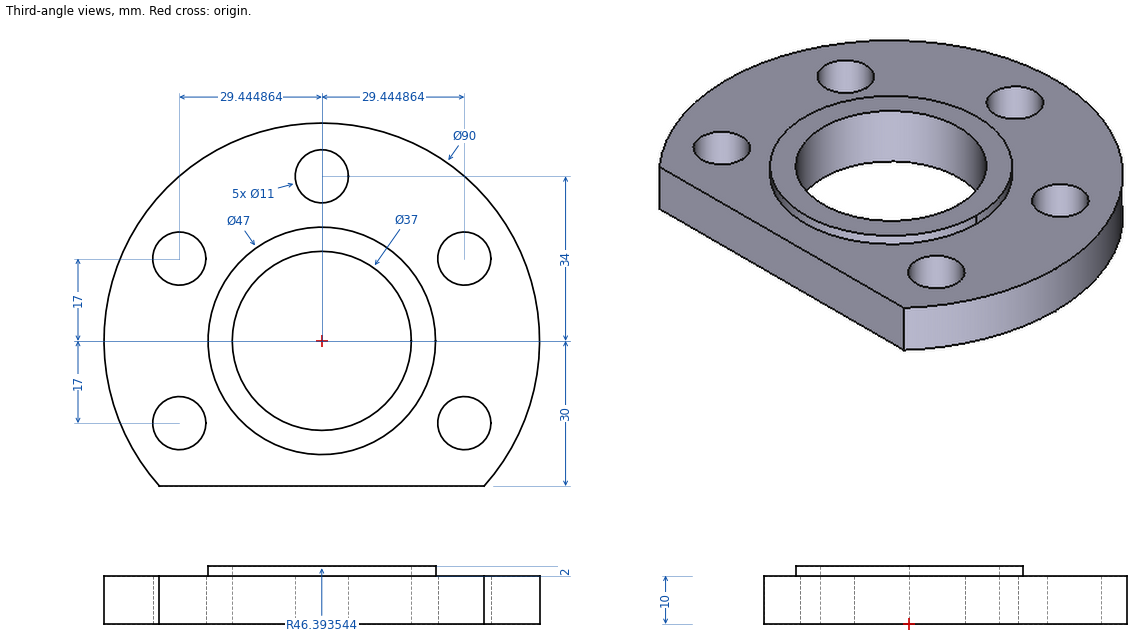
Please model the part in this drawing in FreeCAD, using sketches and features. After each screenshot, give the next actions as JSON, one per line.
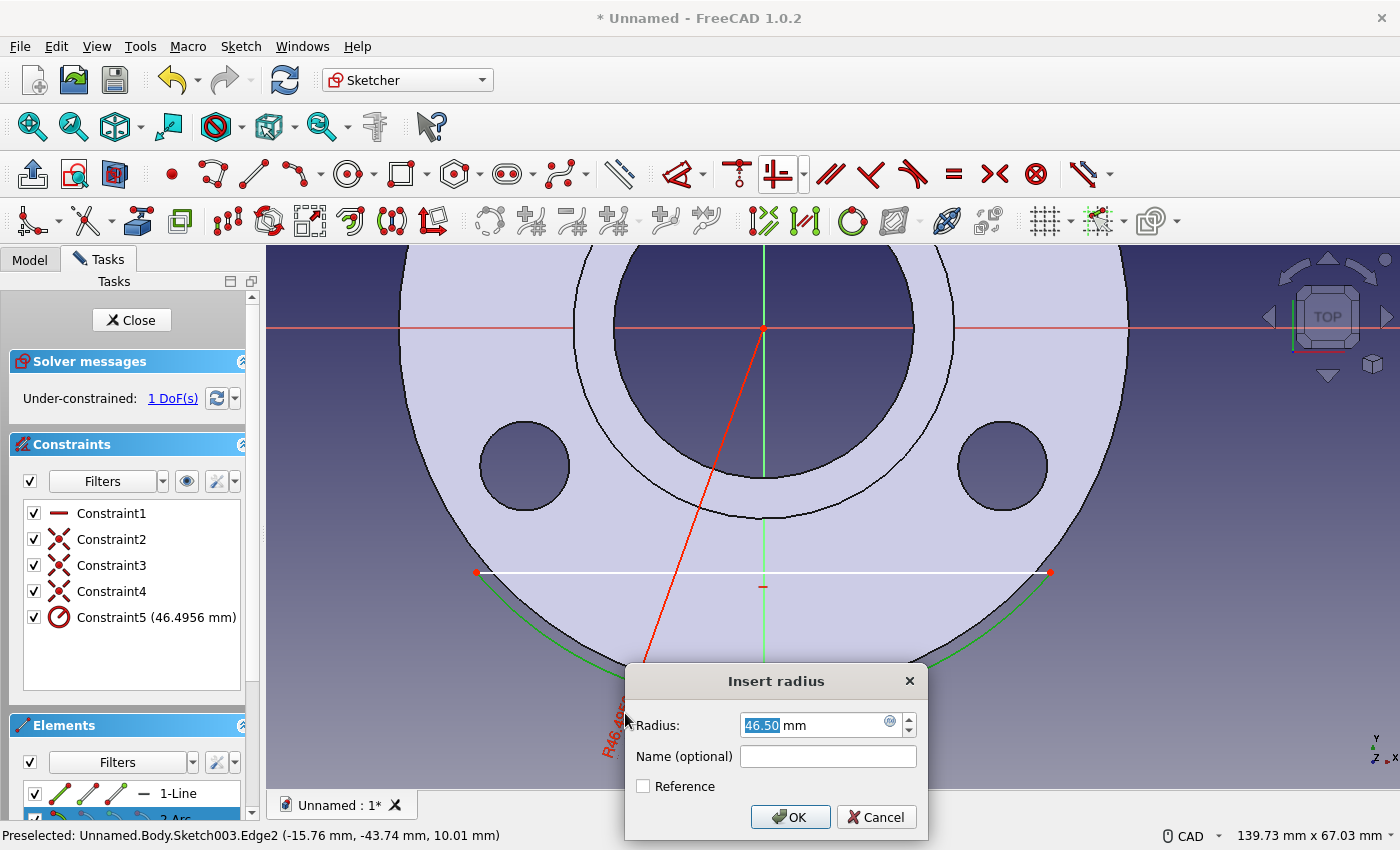
{"action": "type", "text": "46.393544"}
{"action": "key", "text": "Return"}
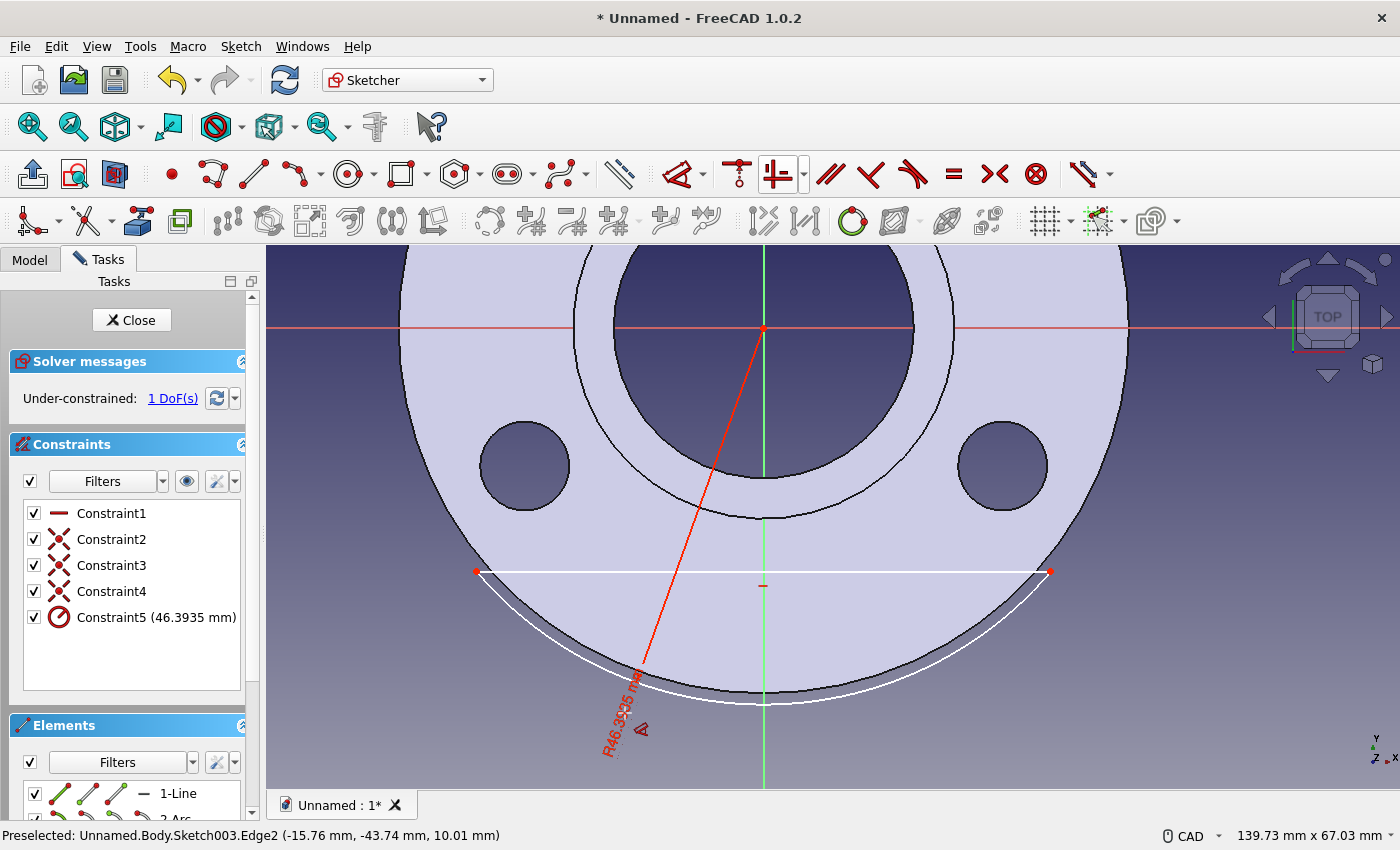
{"action": "left_click", "coordinate": [1051, 572]}
{"action": "left_click", "coordinate": [1085, 450]}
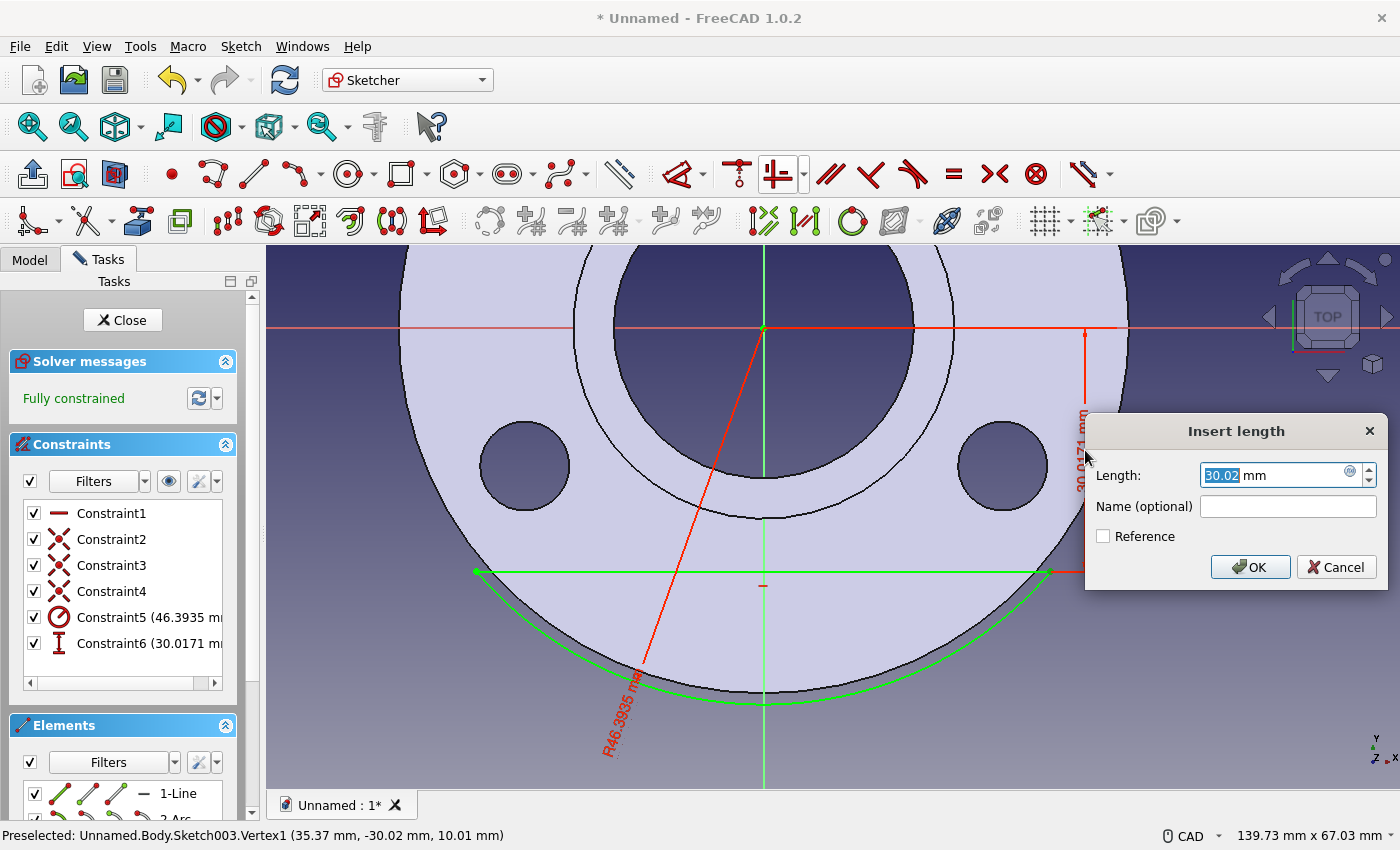
{"action": "type", "text": "30"}
{"action": "key", "text": "Return"}
{"action": "key", "text": "Escape"}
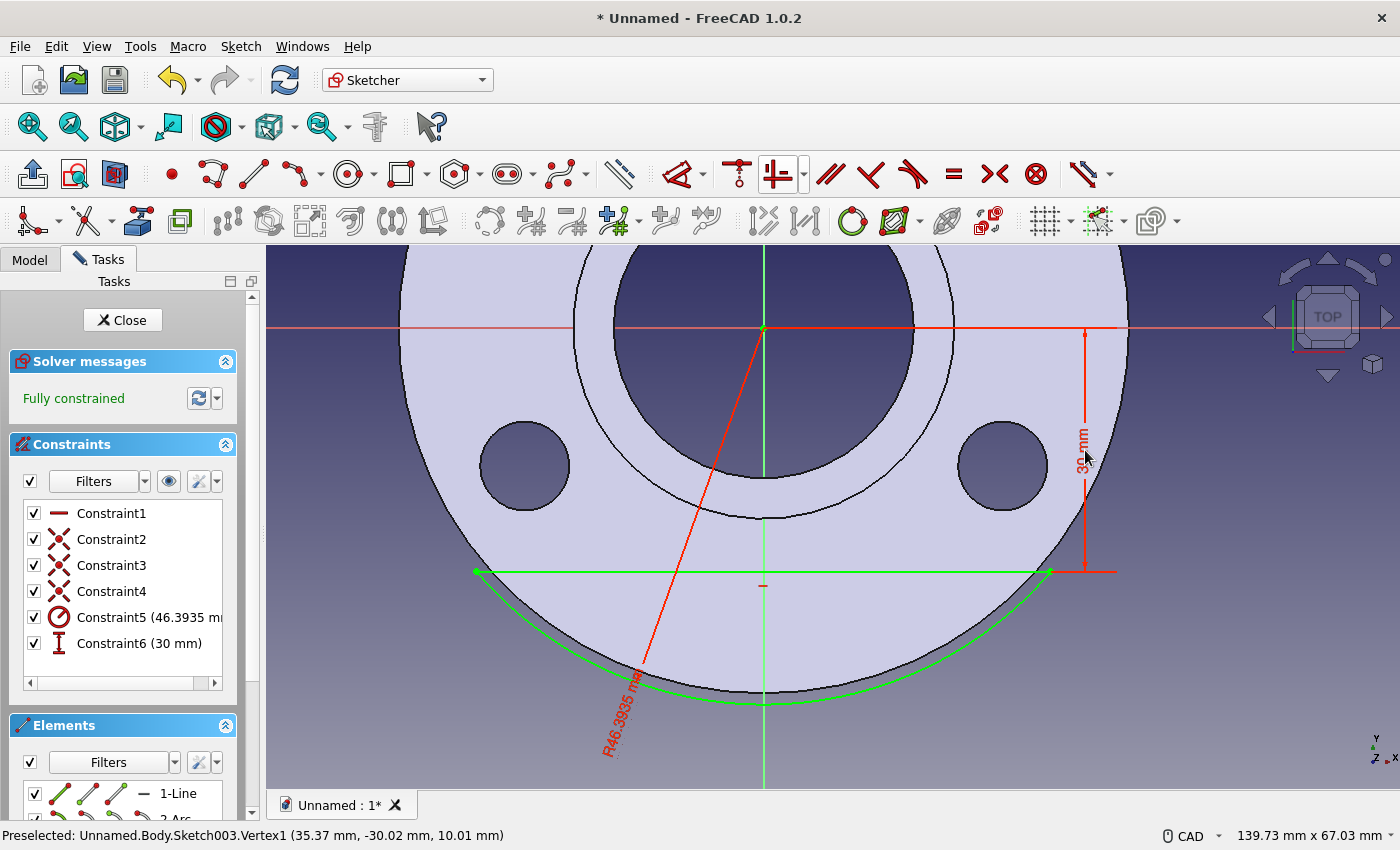
{"action": "left_click", "coordinate": [123, 320]}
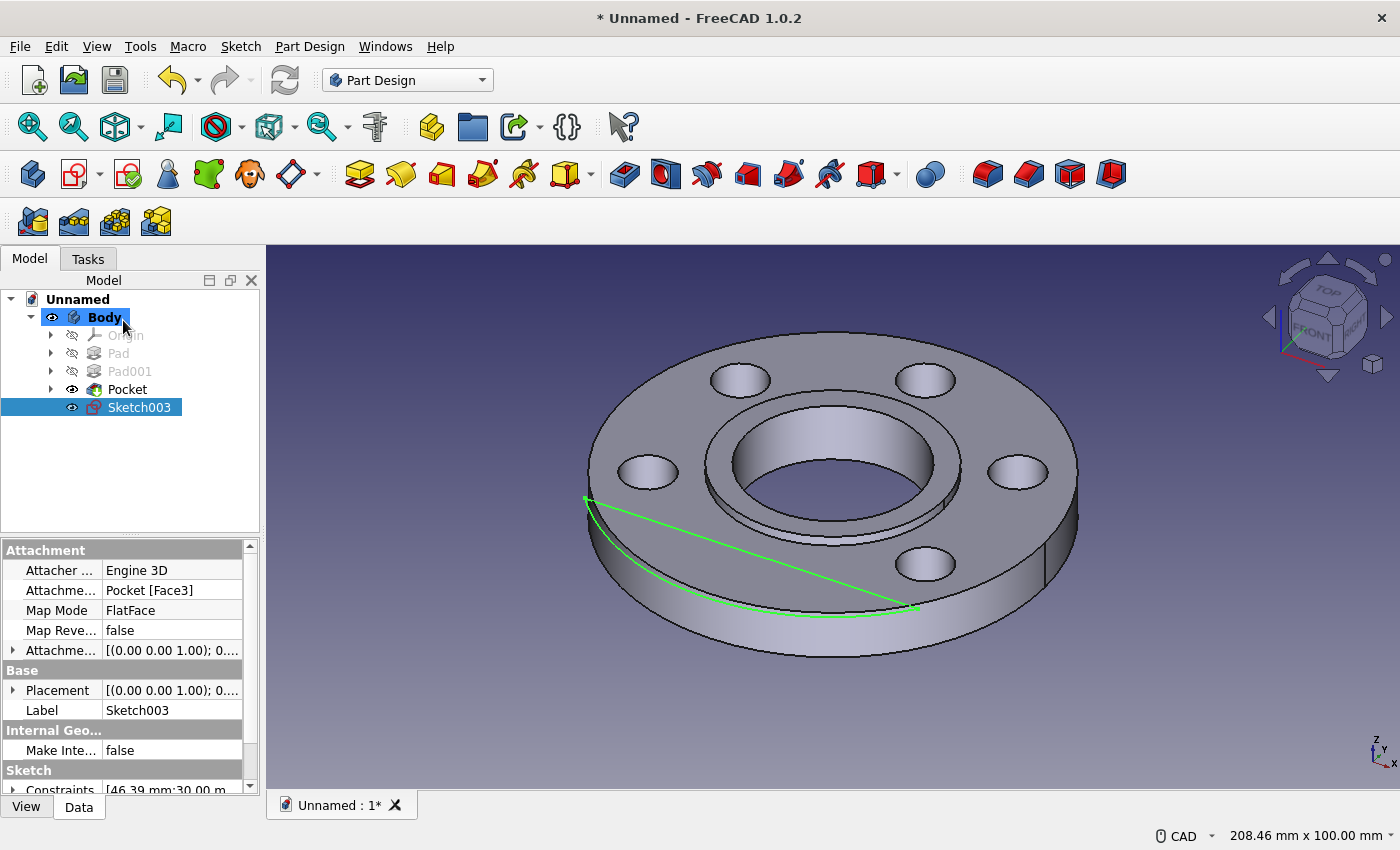
{"action": "left_click", "coordinate": [625, 174]}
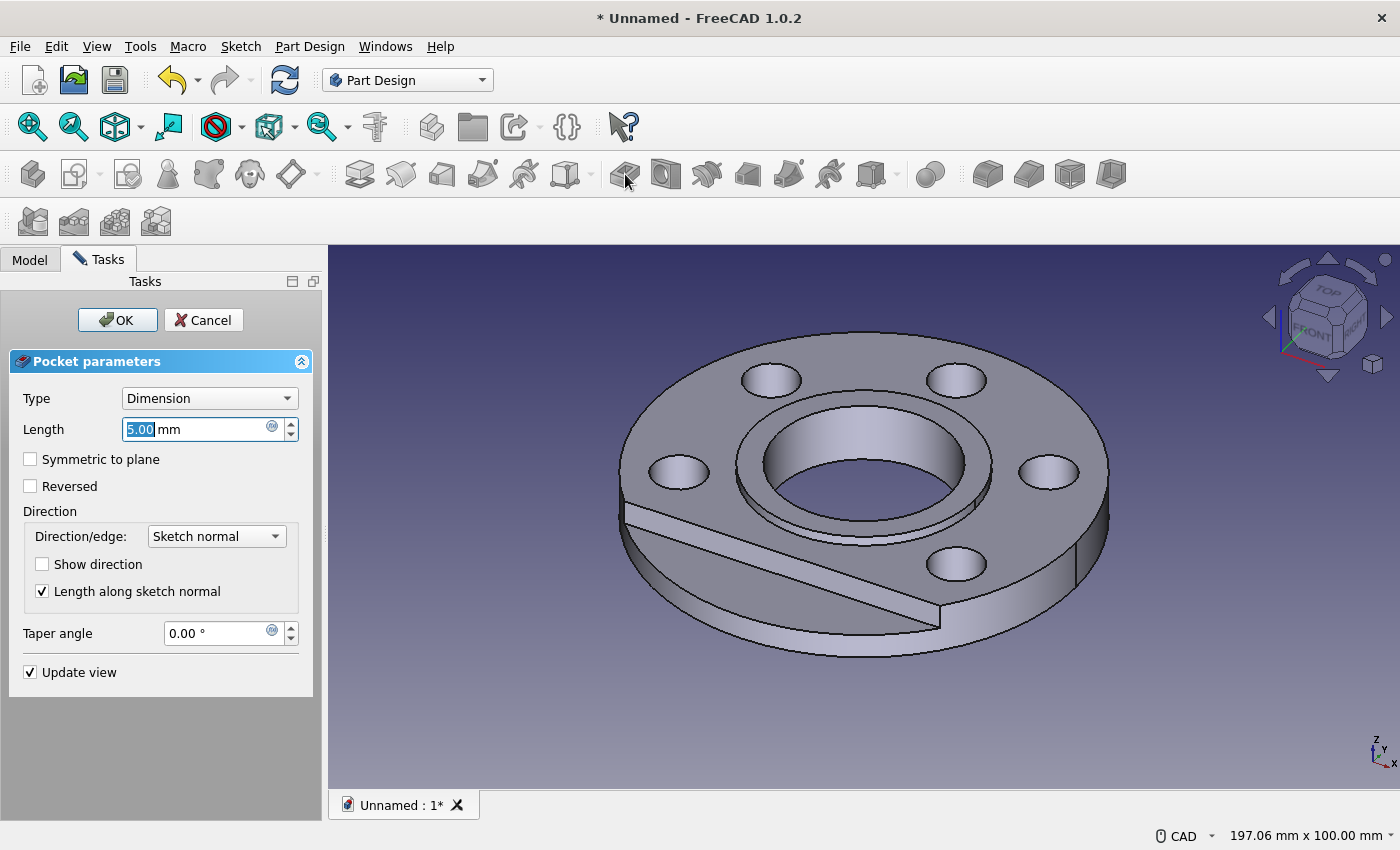
{"action": "left_click", "coordinate": [210, 398]}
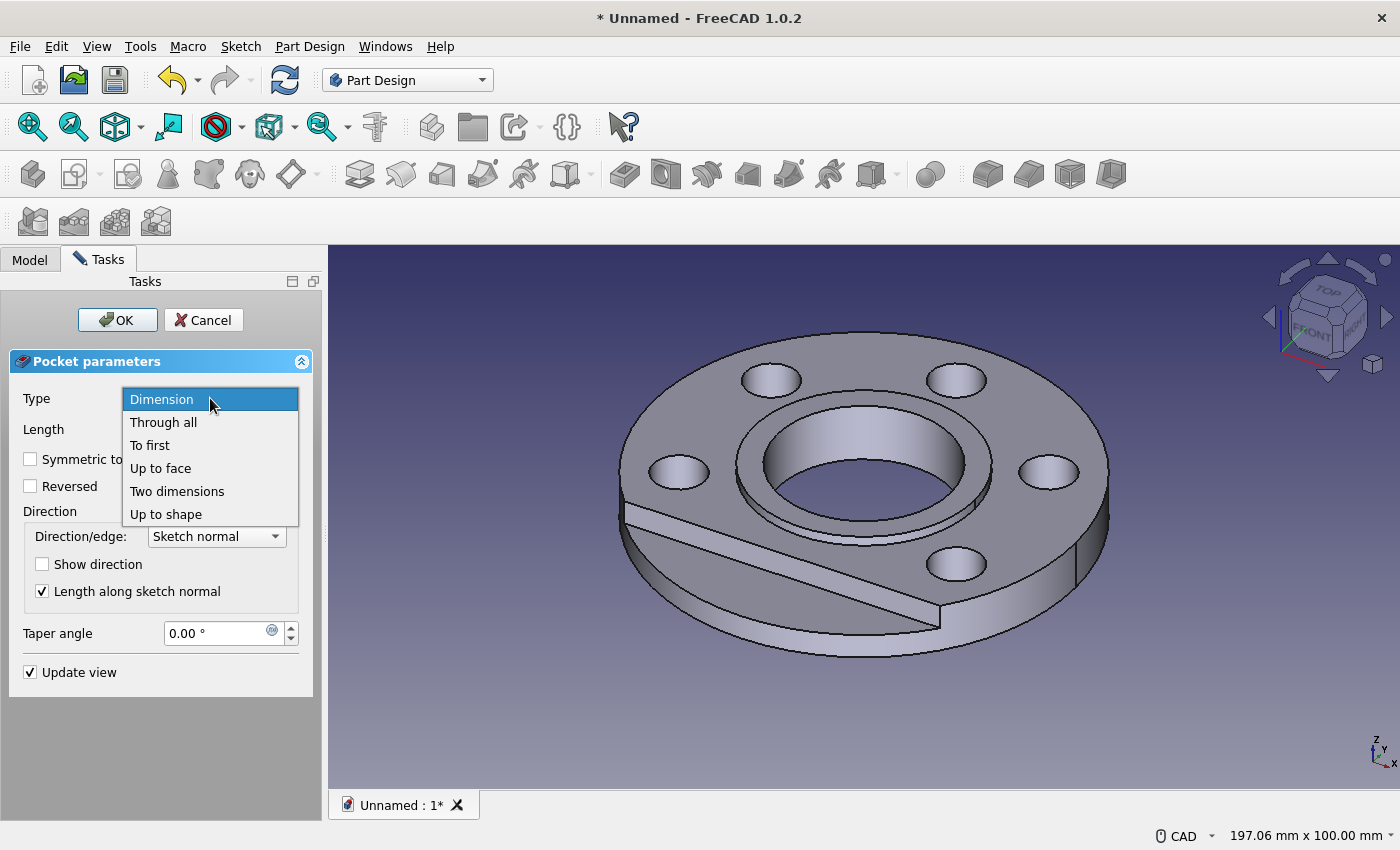
{"action": "left_click", "coordinate": [208, 422]}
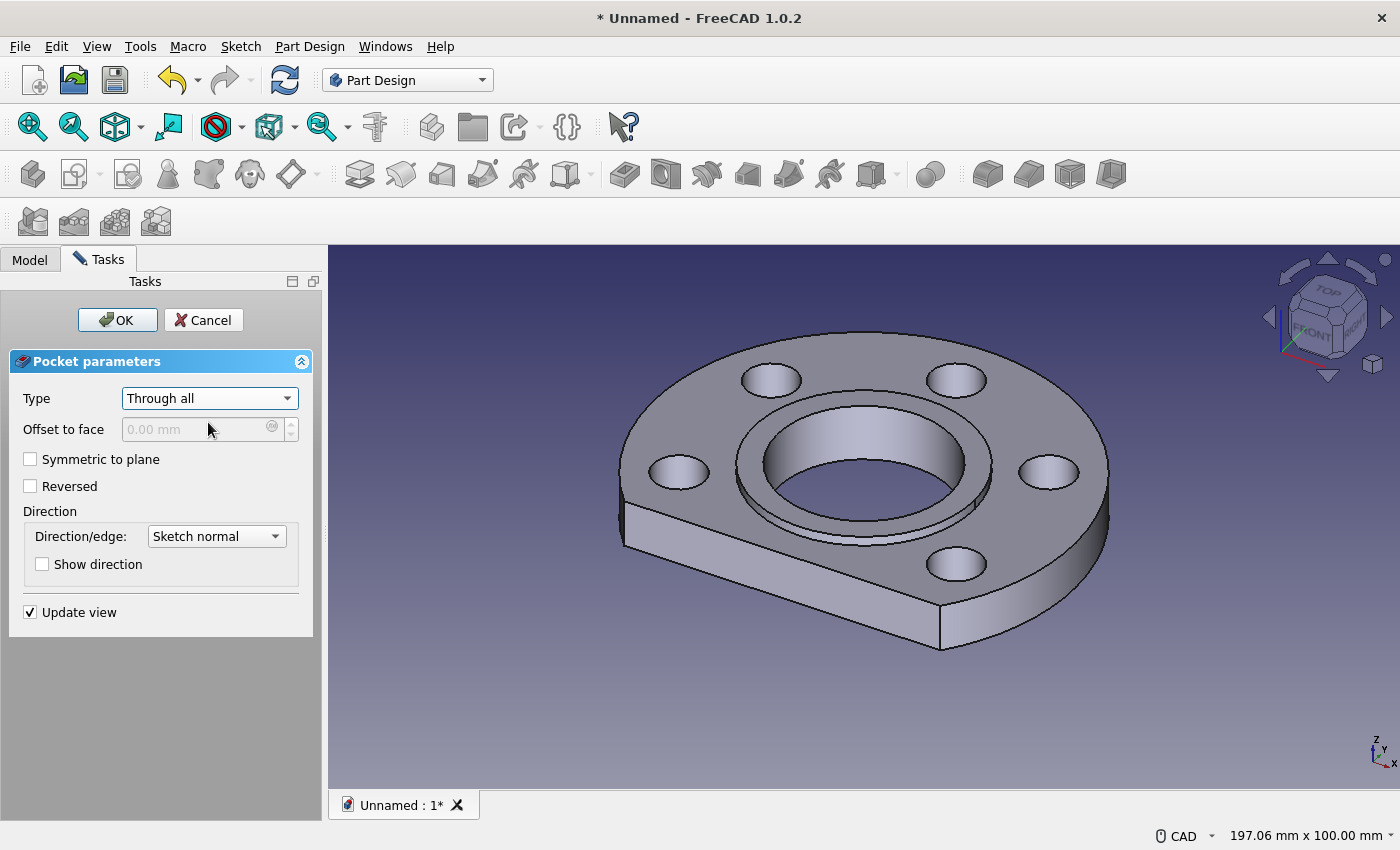
{"action": "left_click", "coordinate": [118, 320]}